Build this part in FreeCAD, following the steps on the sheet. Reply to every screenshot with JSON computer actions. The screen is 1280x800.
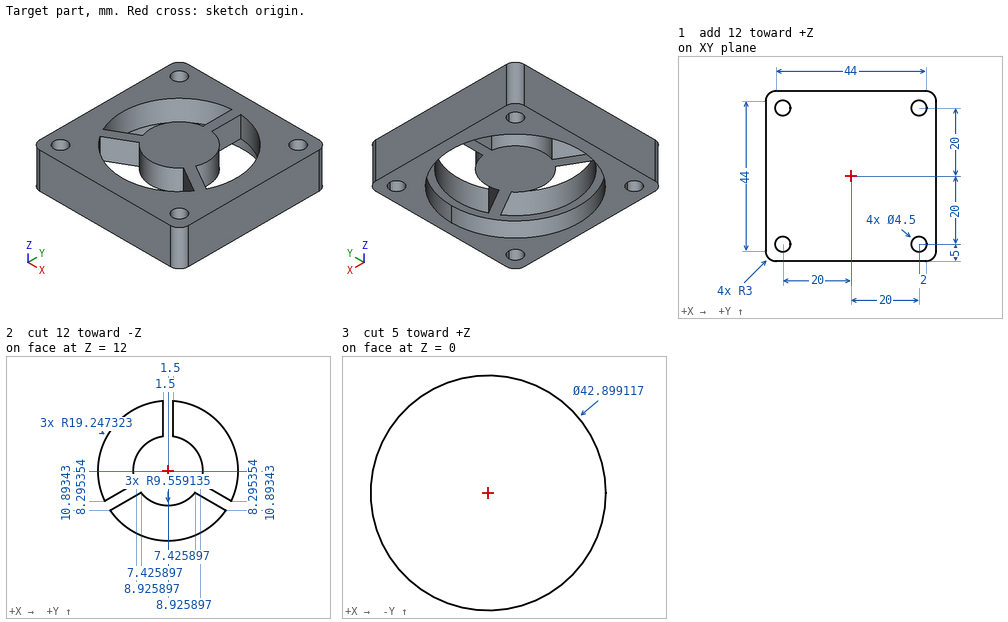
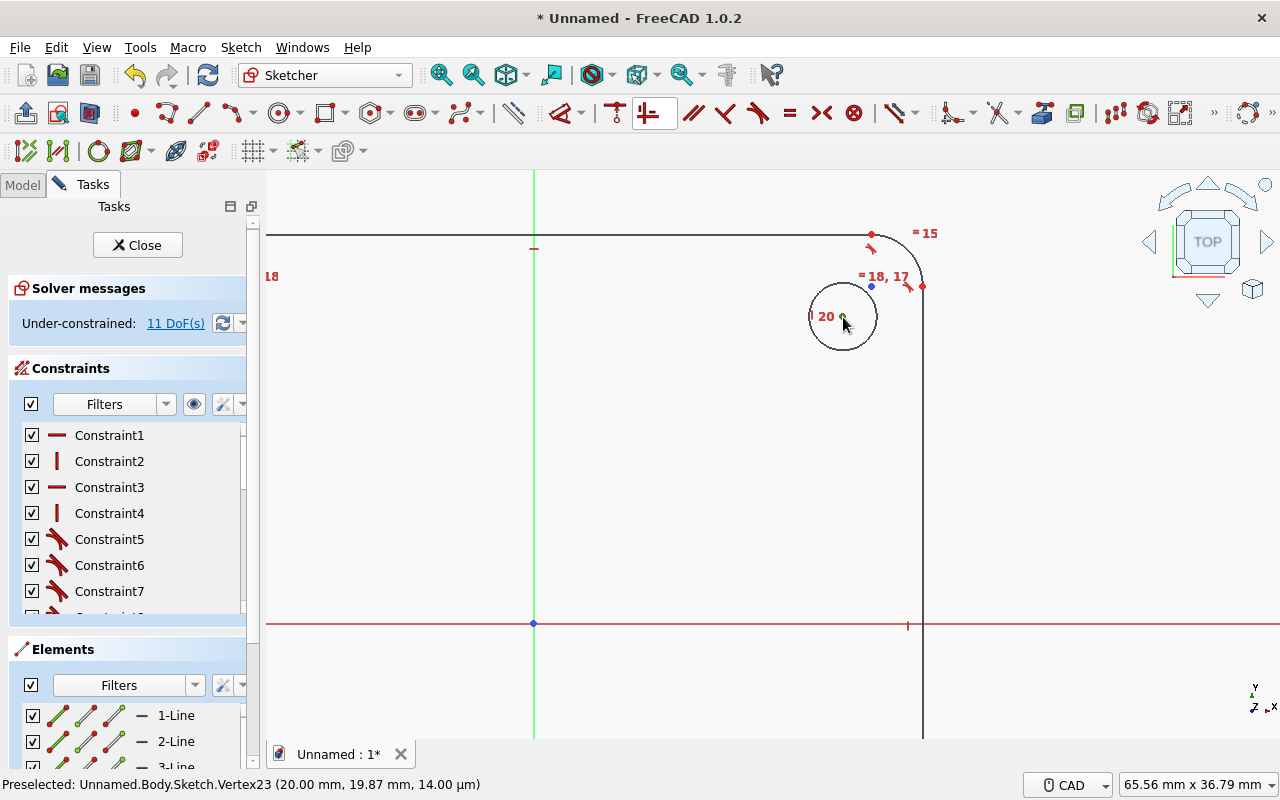
{"action": "scroll", "coordinate": [844, 316], "scroll_direction": "down", "scroll_amount": 4}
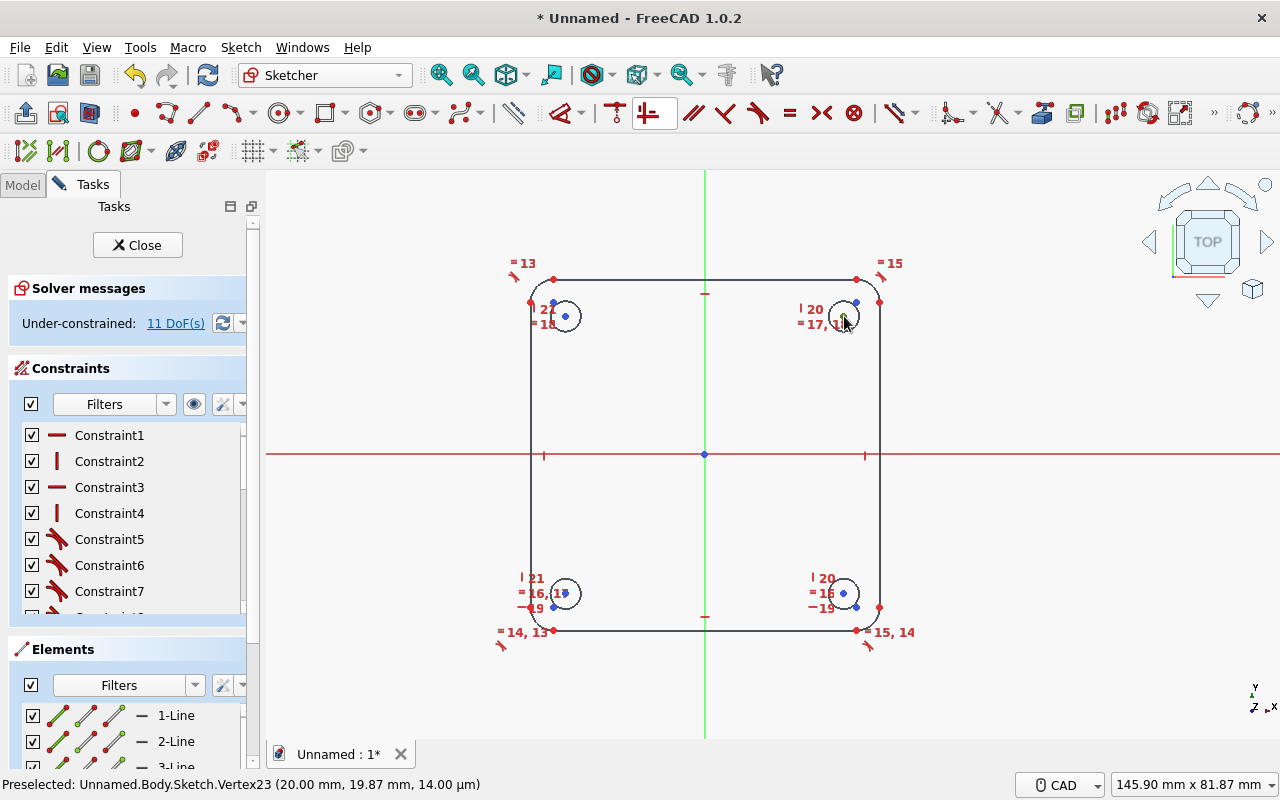
{"action": "left_click", "coordinate": [566, 316]}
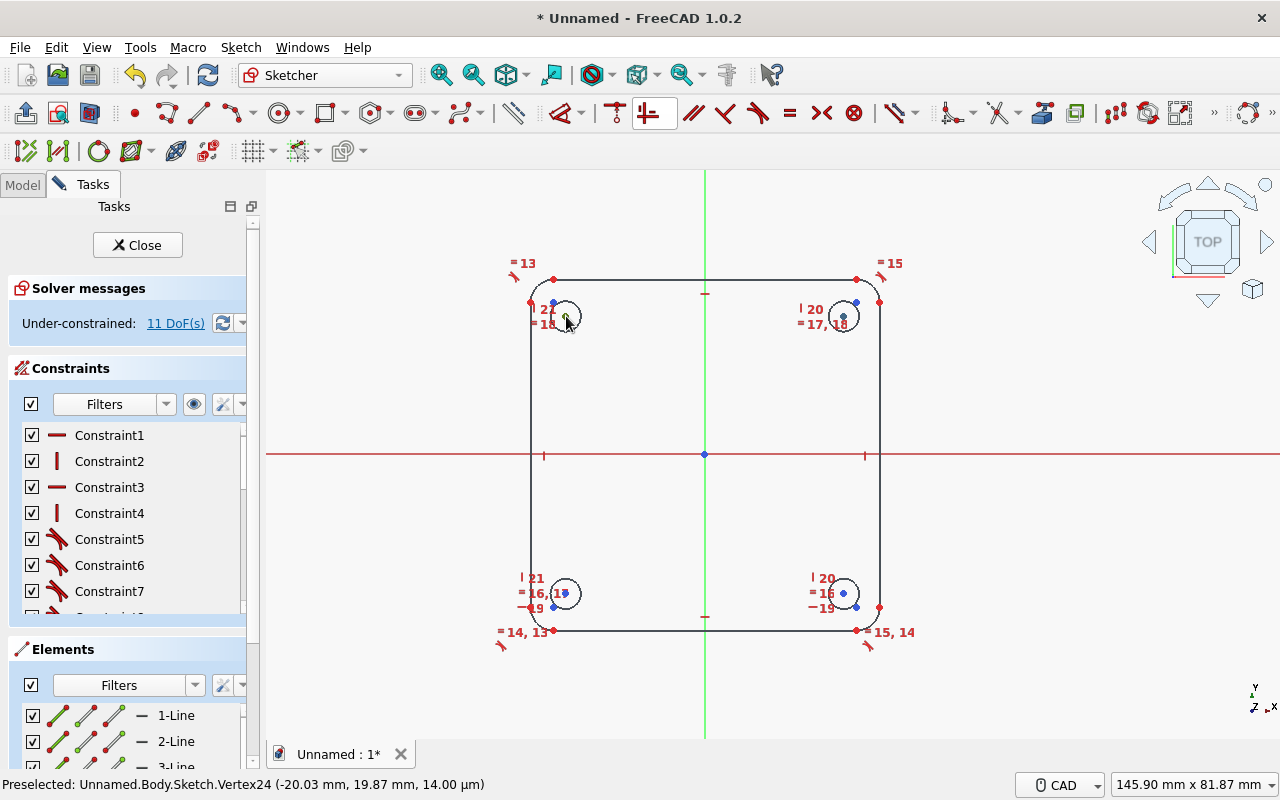
{"action": "left_click", "coordinate": [672, 114]}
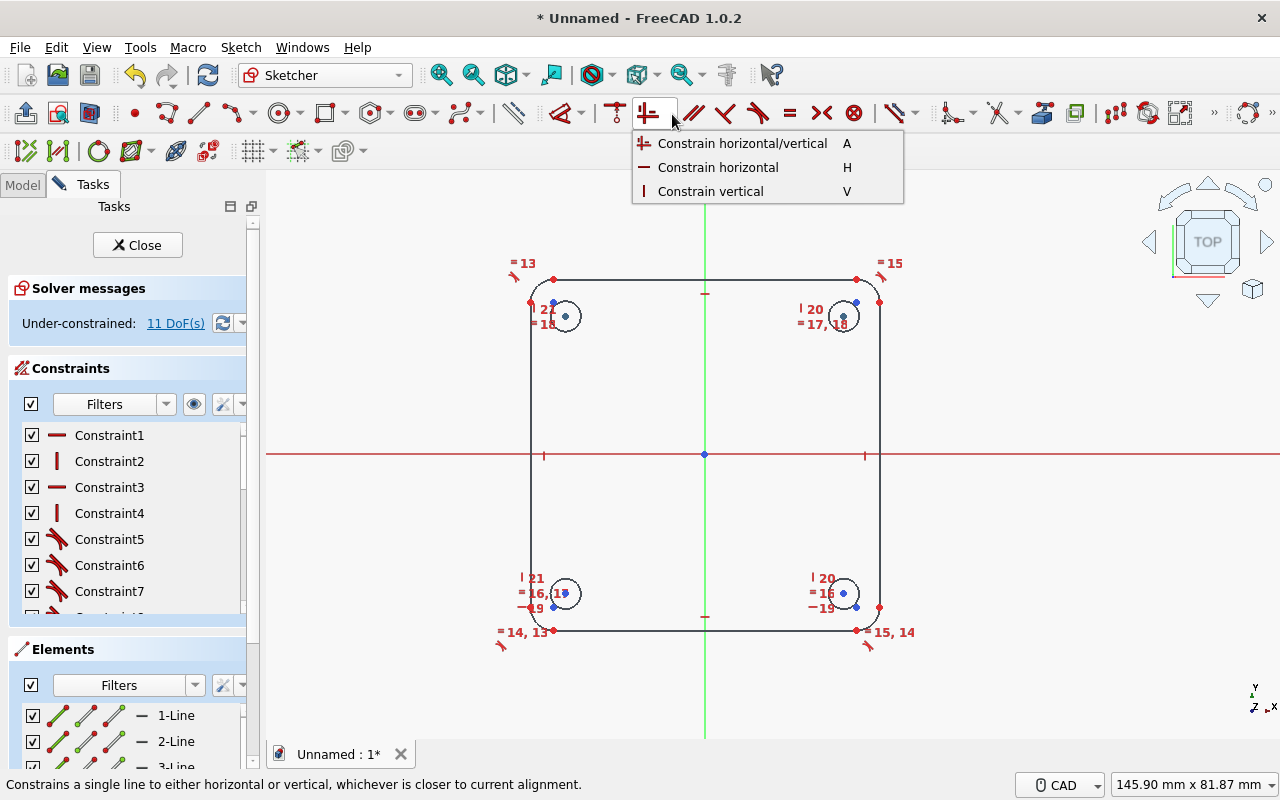
{"action": "left_click", "coordinate": [768, 167]}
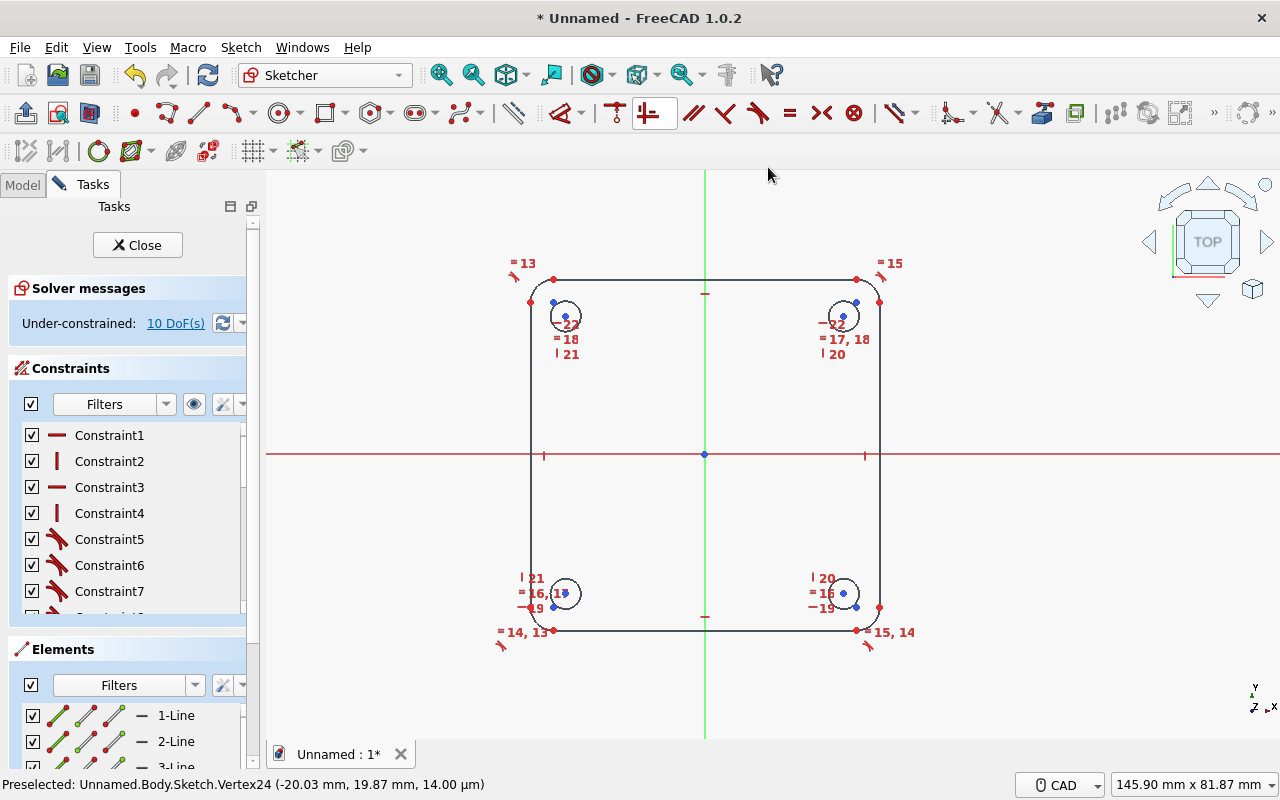
{"action": "left_click", "coordinate": [560, 114]}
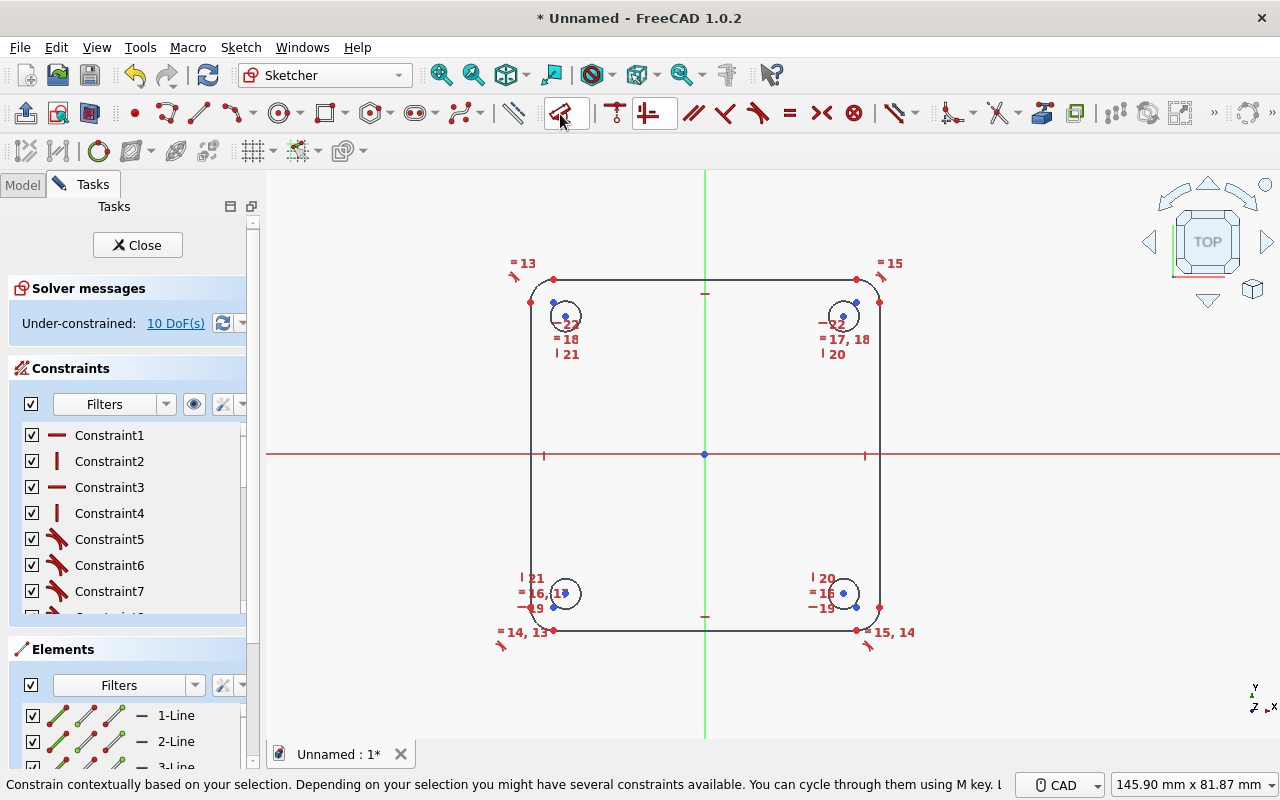
{"action": "scroll", "coordinate": [543, 282], "scroll_direction": "up", "scroll_amount": 4}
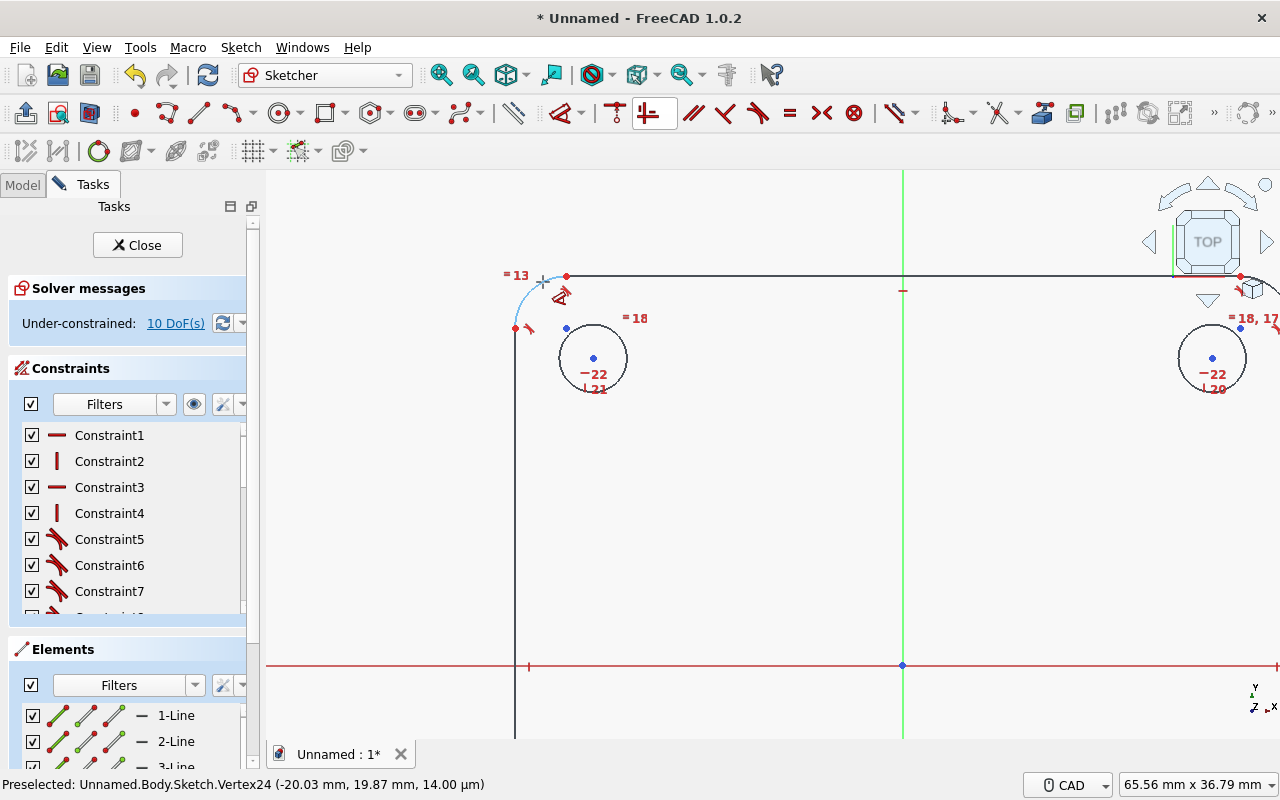
{"action": "left_click", "coordinate": [543, 282]}
{"action": "left_click", "coordinate": [528, 254]}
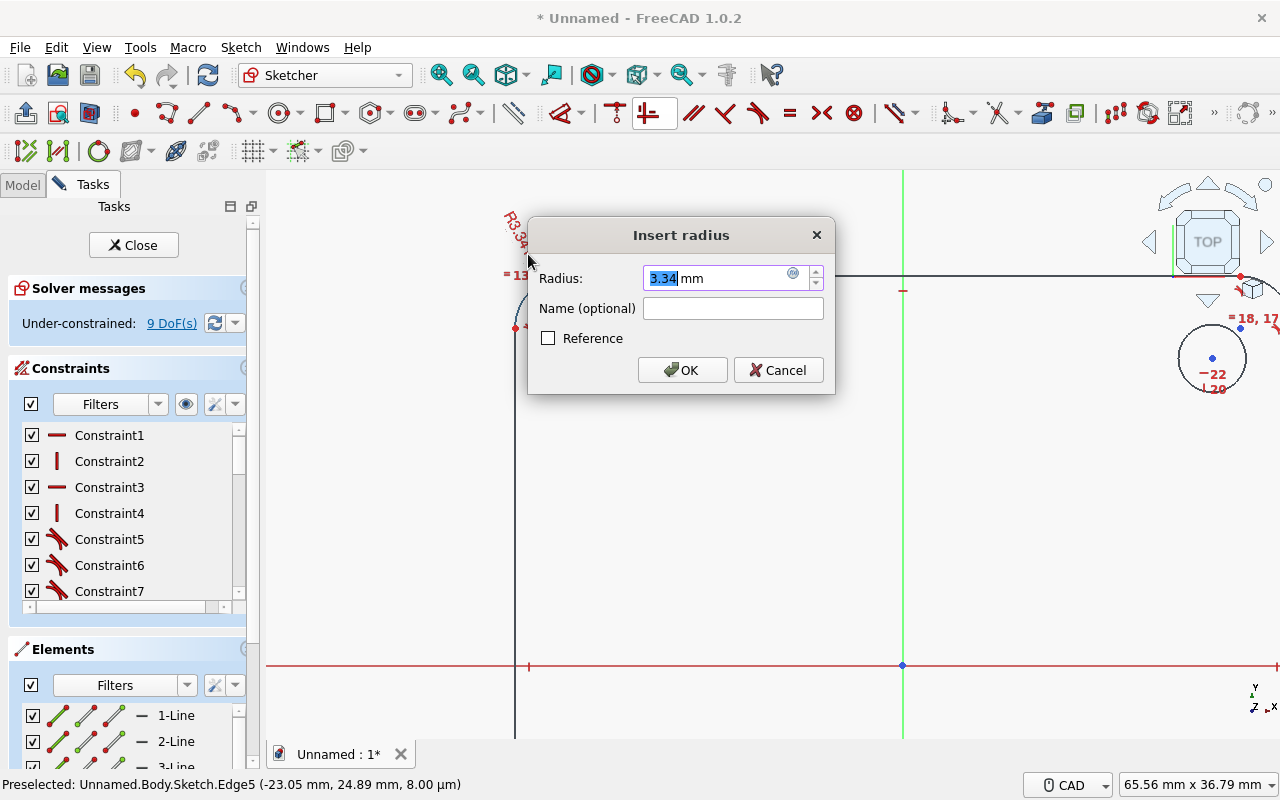
{"action": "type", "text": "3"}
{"action": "key", "text": "Return"}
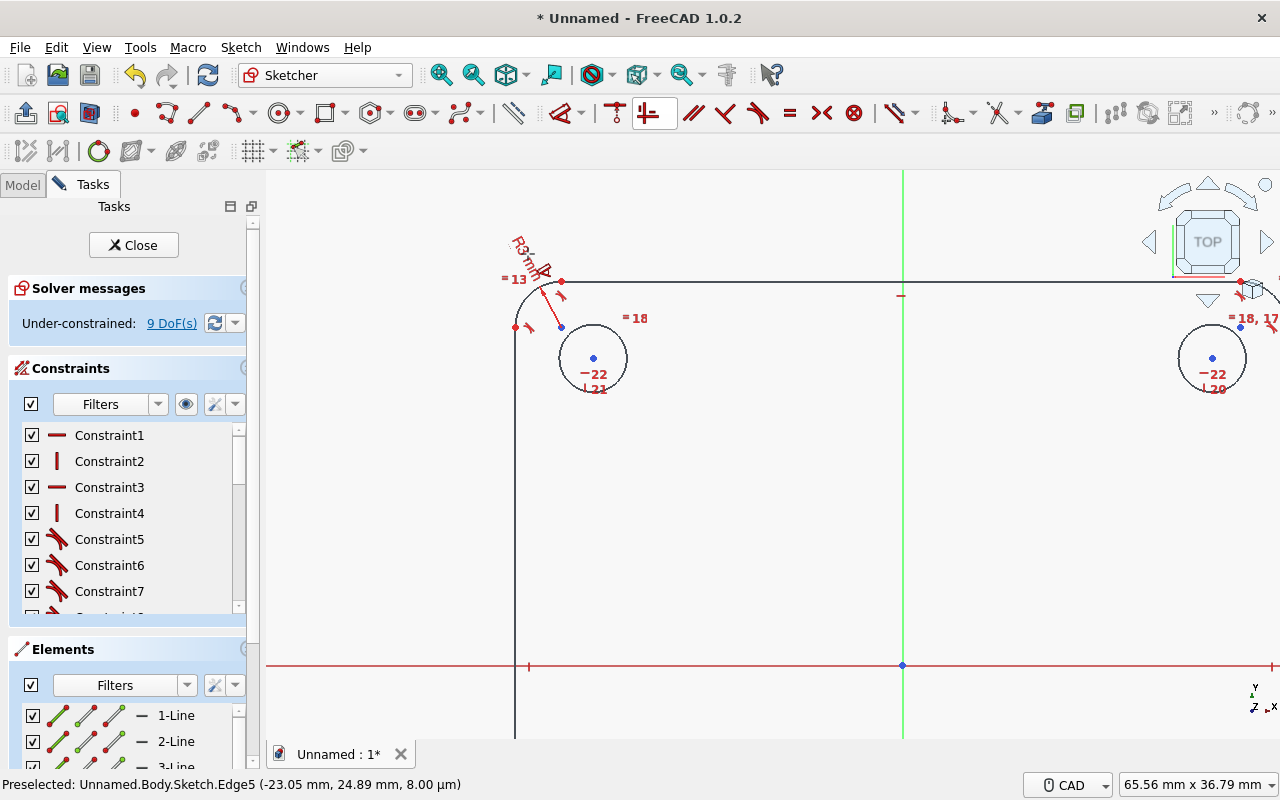
{"action": "scroll", "coordinate": [543, 282], "scroll_direction": "down", "scroll_amount": 4}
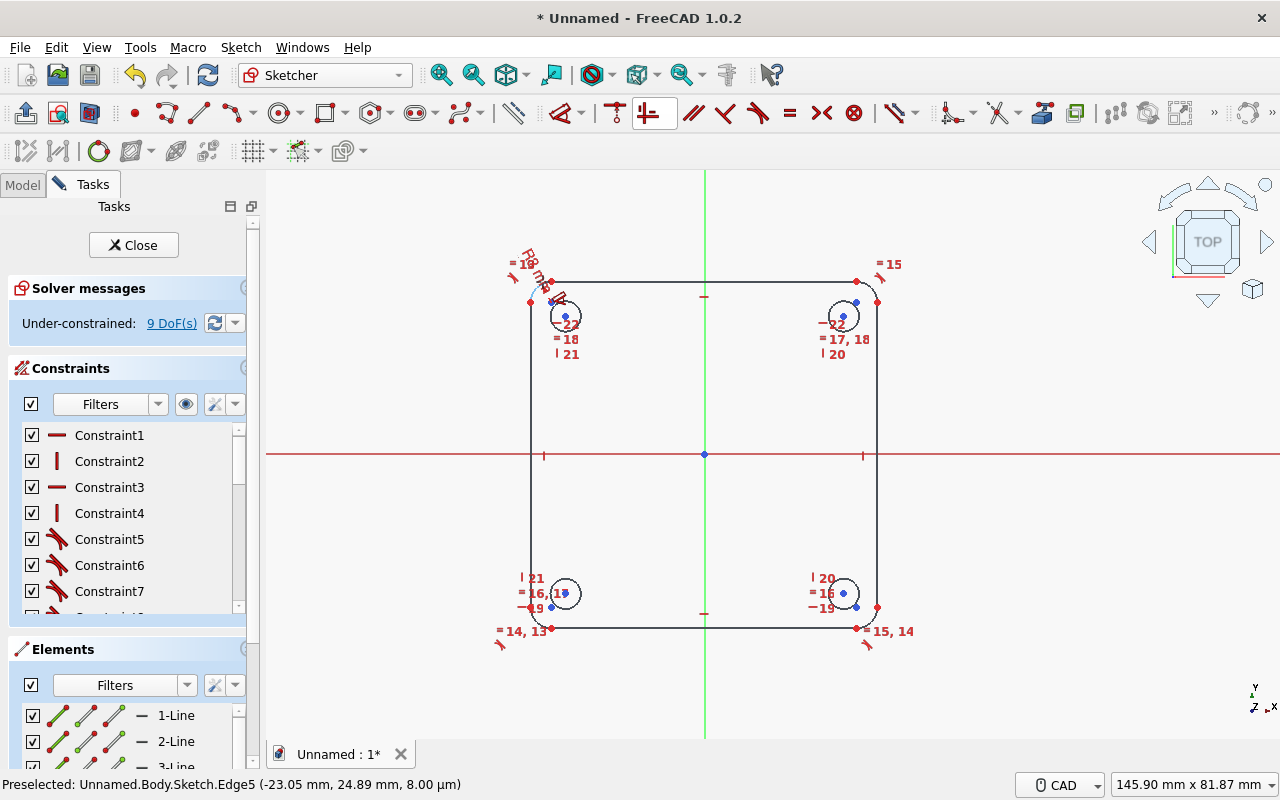
{"action": "scroll", "coordinate": [855, 583], "scroll_direction": "up", "scroll_amount": 2}